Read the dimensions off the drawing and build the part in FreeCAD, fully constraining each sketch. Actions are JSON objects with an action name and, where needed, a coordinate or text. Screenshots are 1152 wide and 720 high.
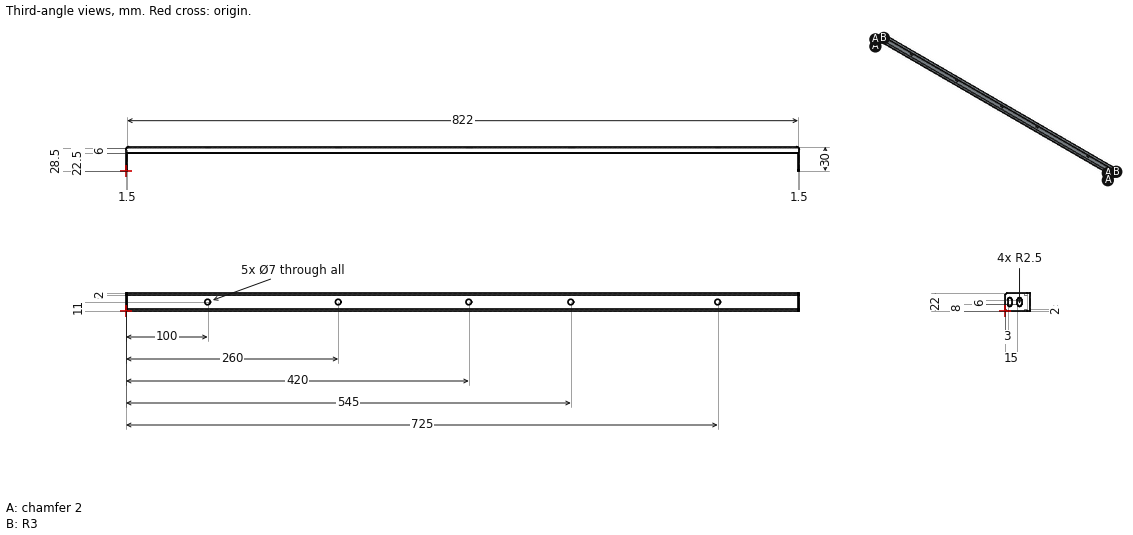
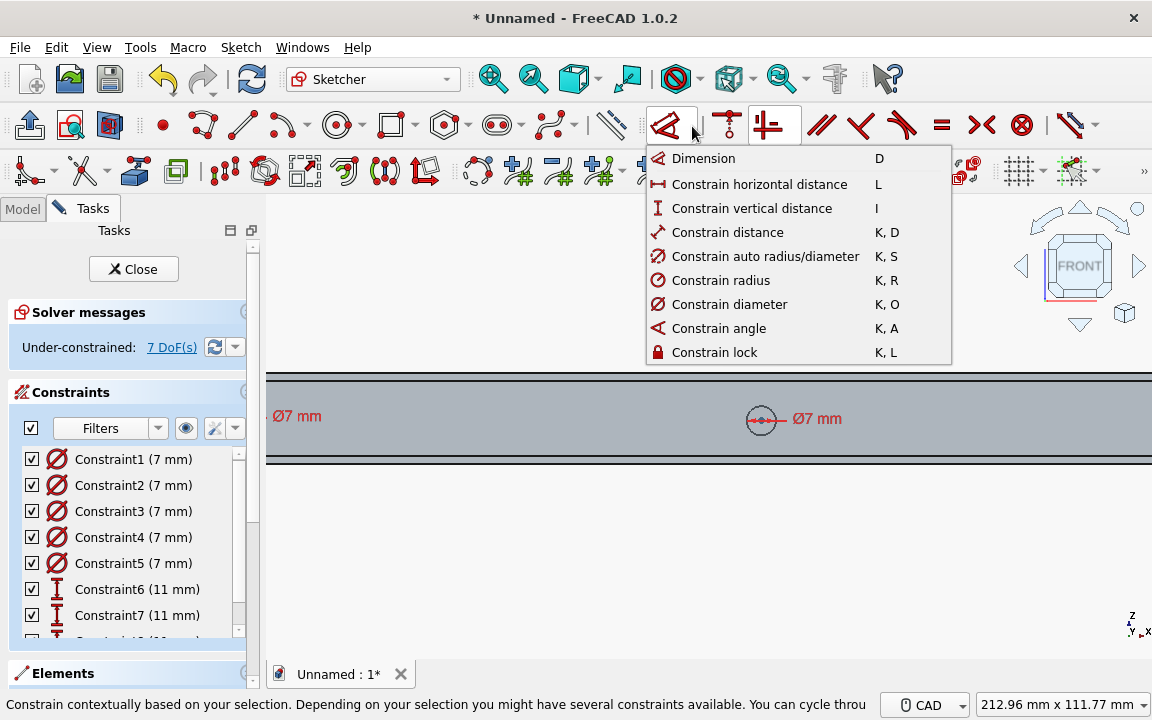
{"action": "left_click", "coordinate": [799, 208]}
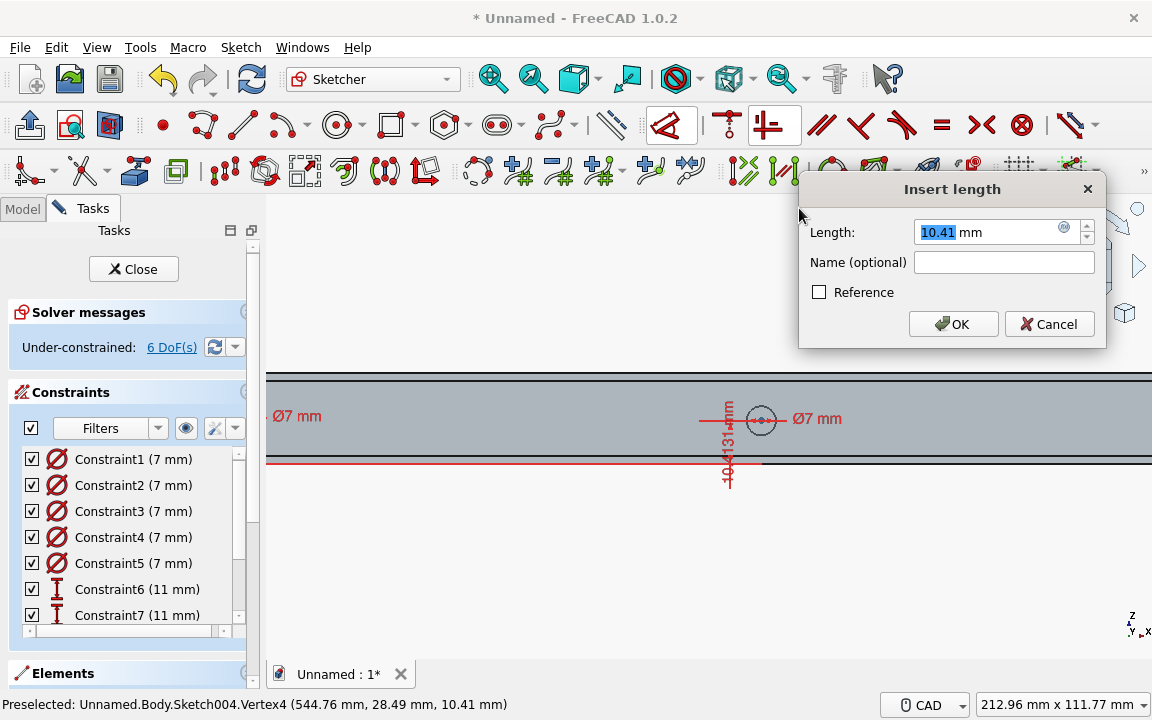
{"action": "type", "text": "11"}
{"action": "key", "text": "Return"}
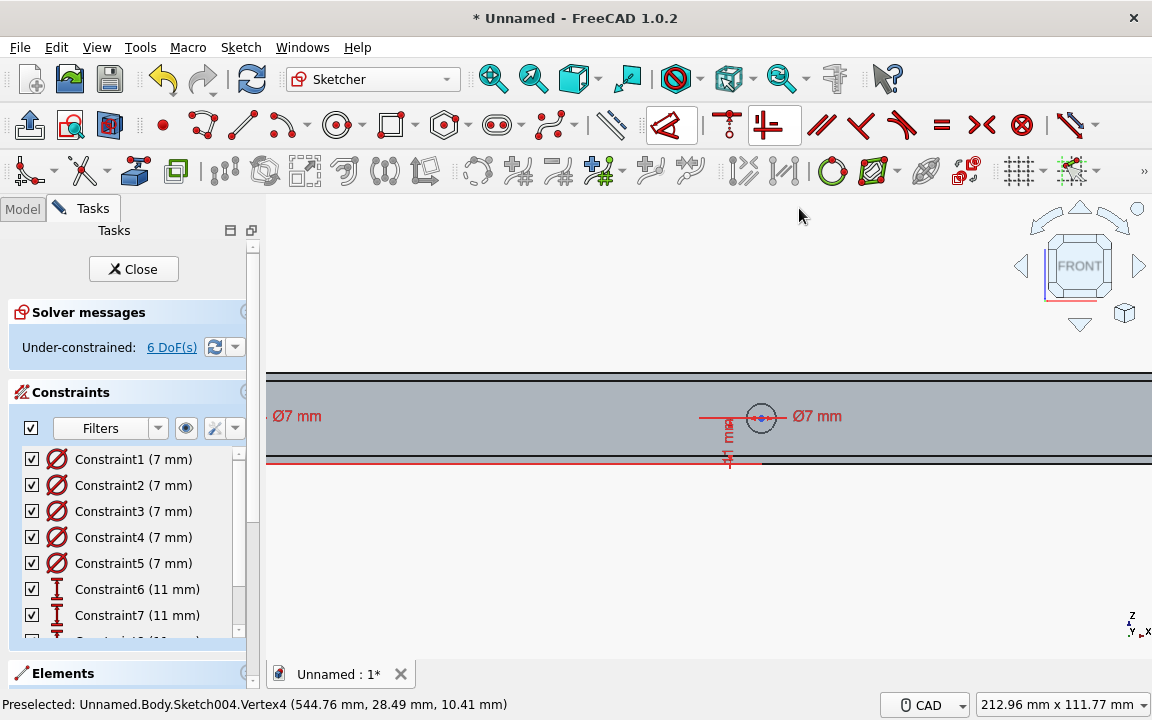
{"action": "scroll", "coordinate": [765, 425], "scroll_direction": "down", "scroll_amount": 9}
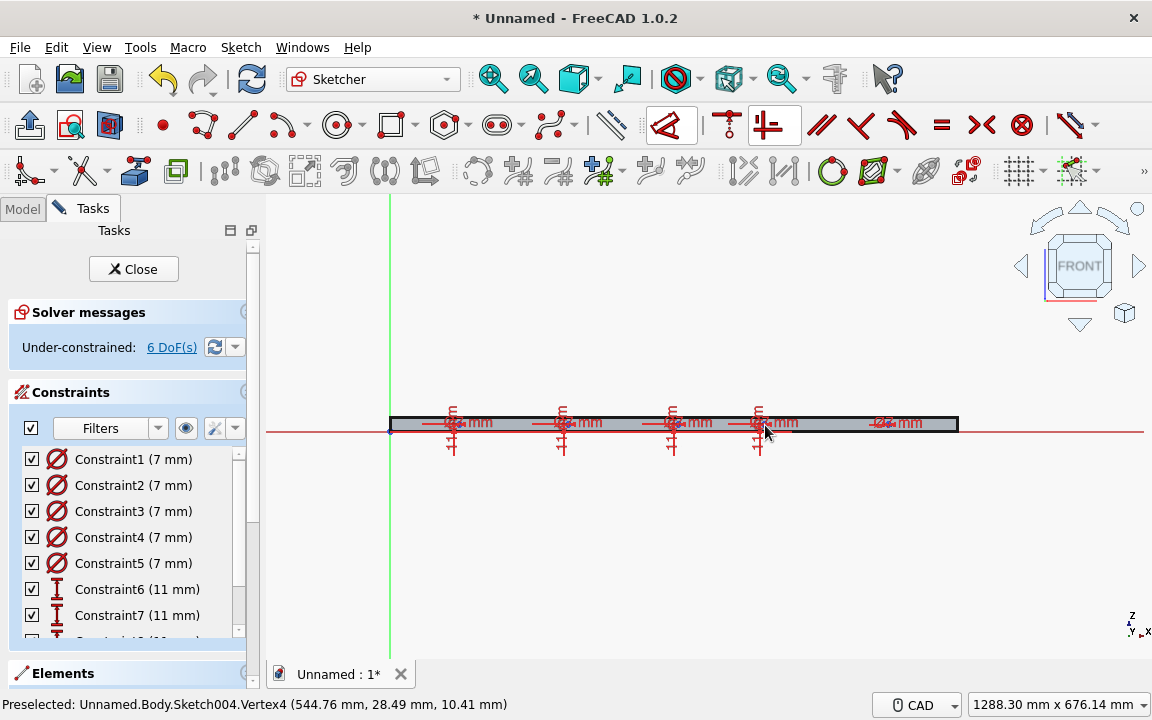
{"action": "scroll", "coordinate": [889, 425], "scroll_direction": "up", "scroll_amount": 9}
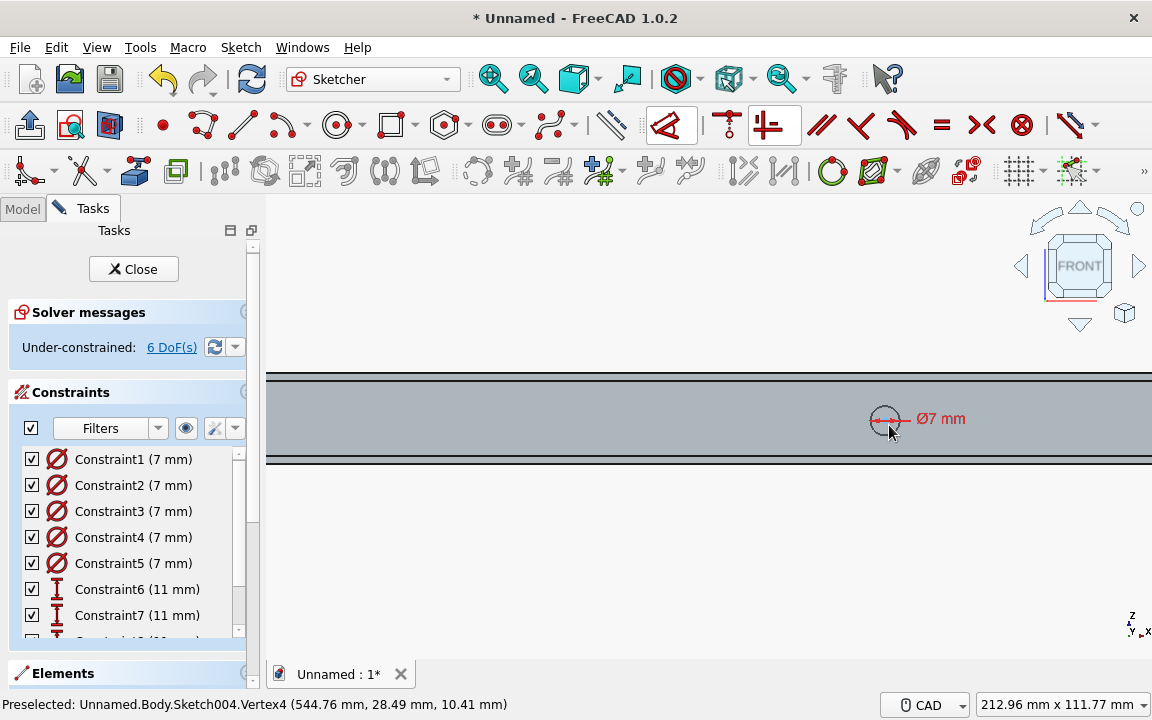
{"action": "left_click", "coordinate": [885, 421]}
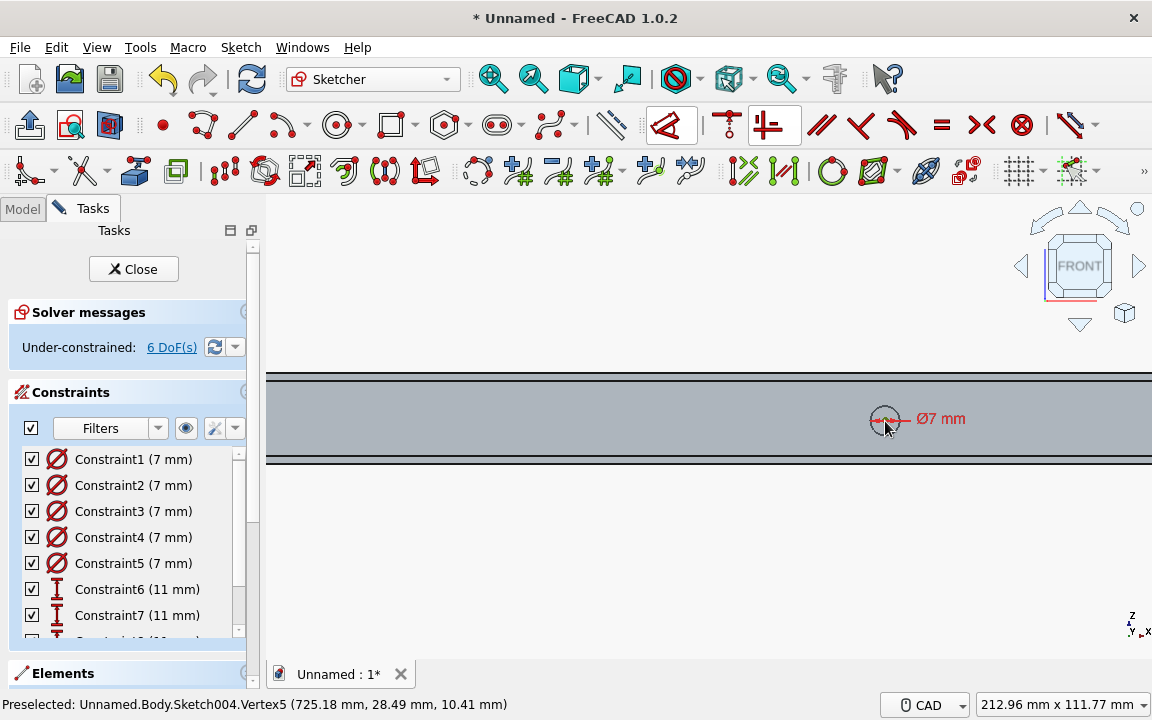
{"action": "key", "text": "i"}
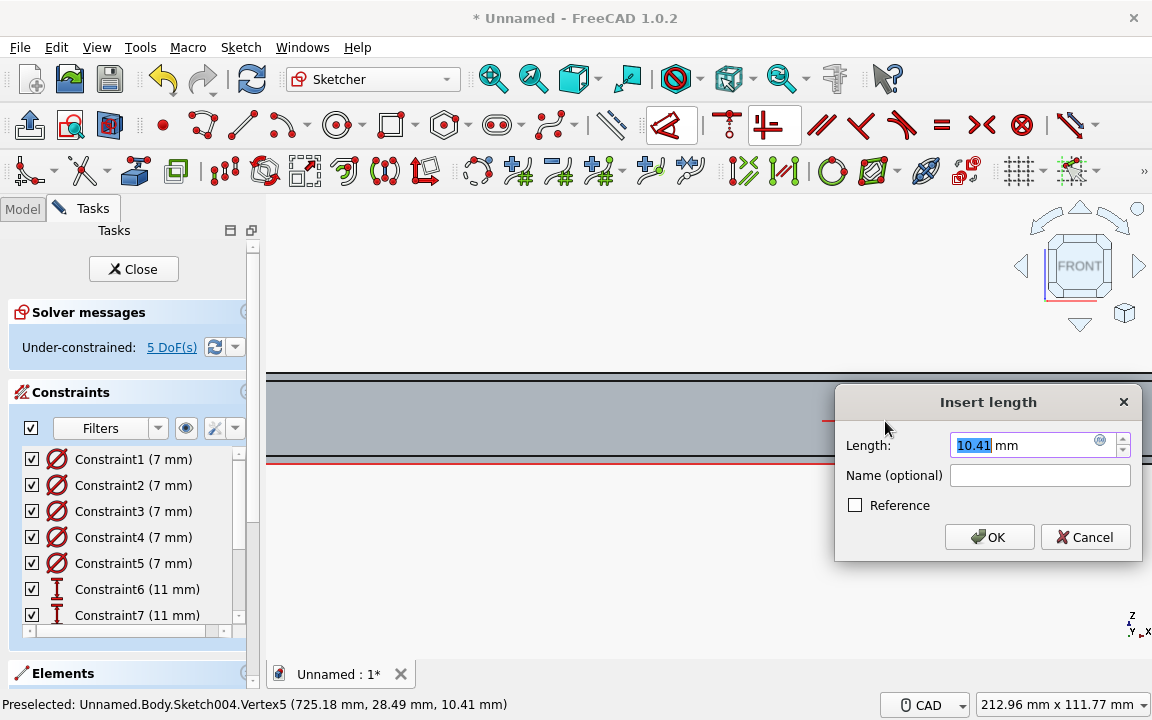
{"action": "type", "text": "11"}
{"action": "key", "text": "Return"}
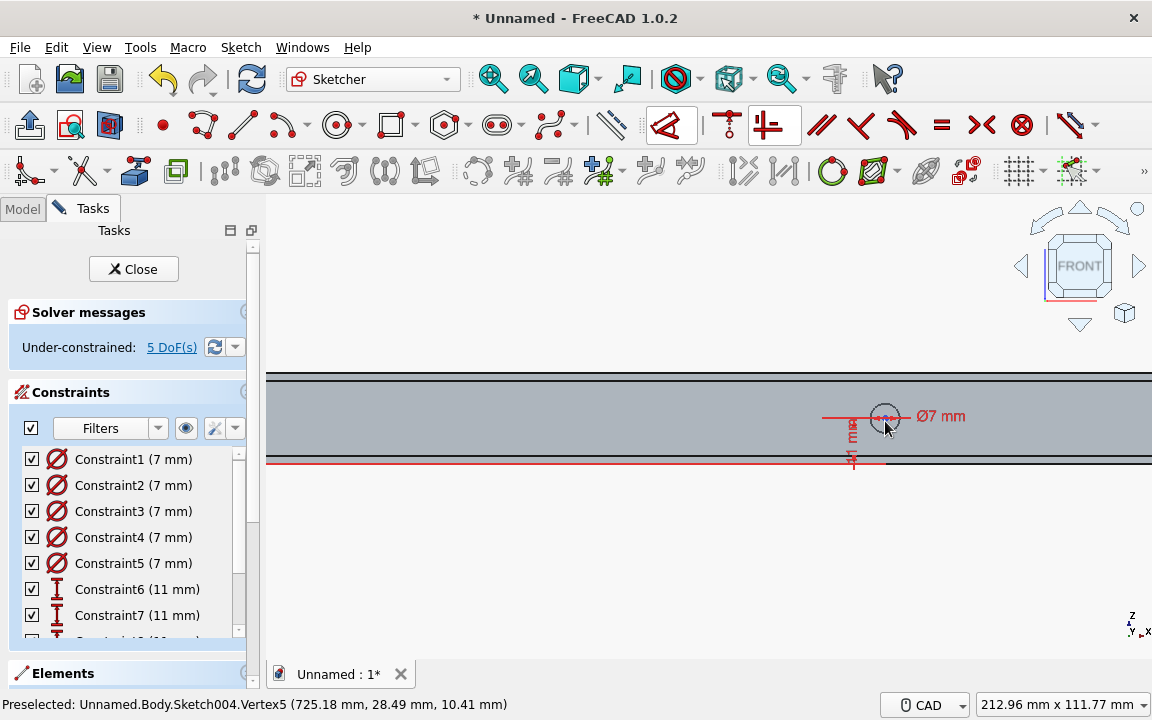
{"action": "scroll", "coordinate": [889, 425], "scroll_direction": "down", "scroll_amount": 9}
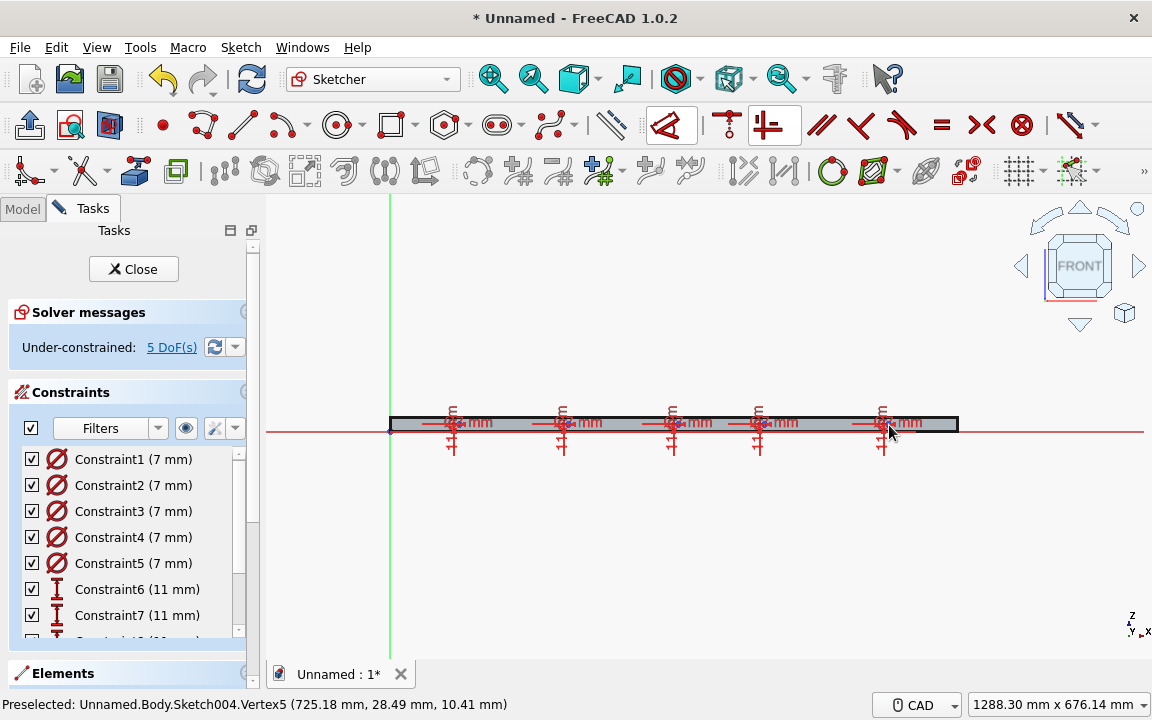
{"action": "left_click", "coordinate": [459, 424]}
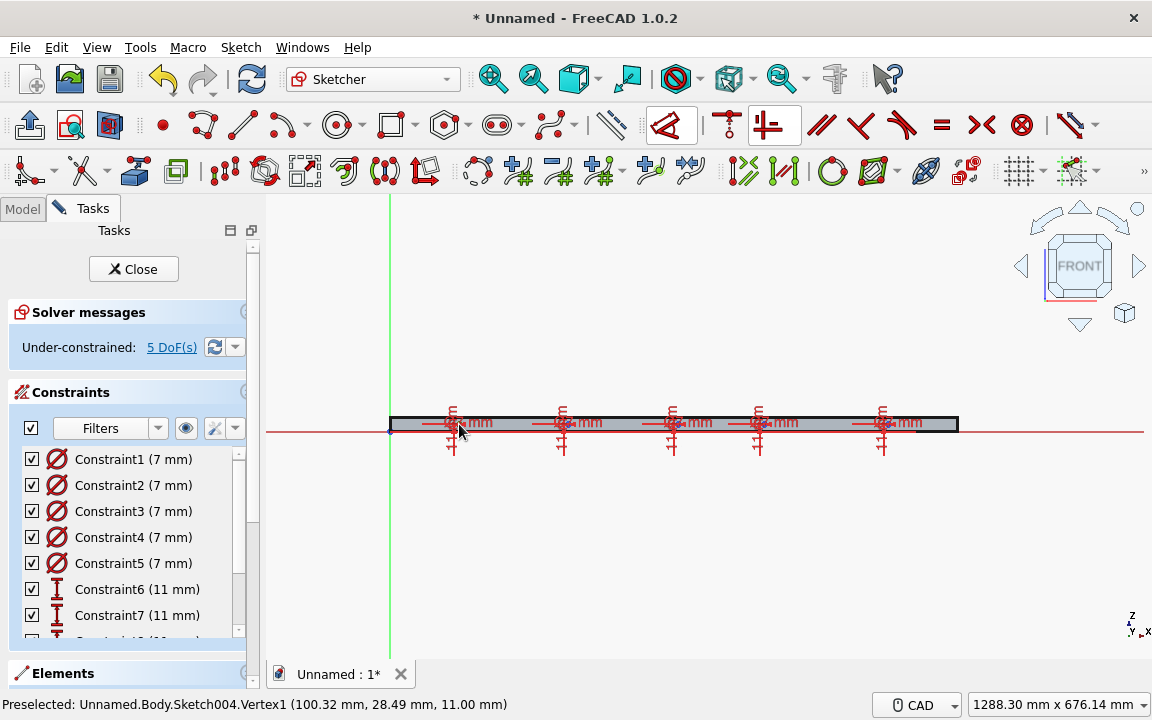
{"action": "left_click", "coordinate": [692, 126]}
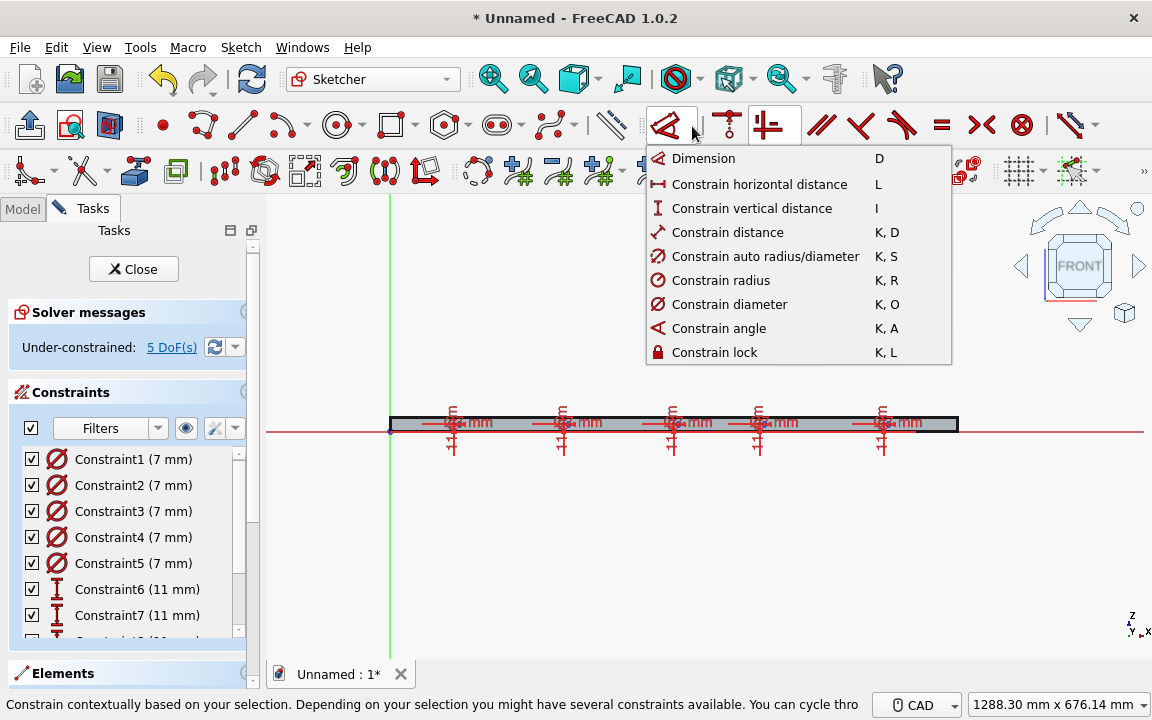
{"action": "left_click", "coordinate": [799, 184]}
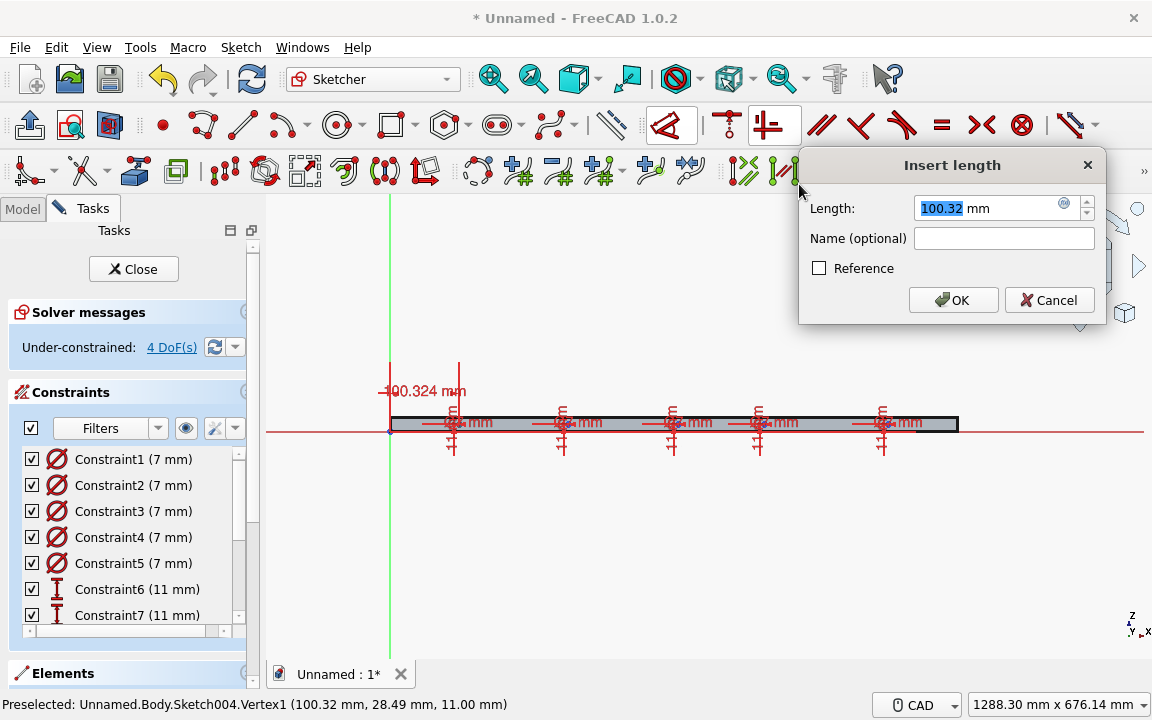
{"action": "type", "text": "100"}
{"action": "key", "text": "Return"}